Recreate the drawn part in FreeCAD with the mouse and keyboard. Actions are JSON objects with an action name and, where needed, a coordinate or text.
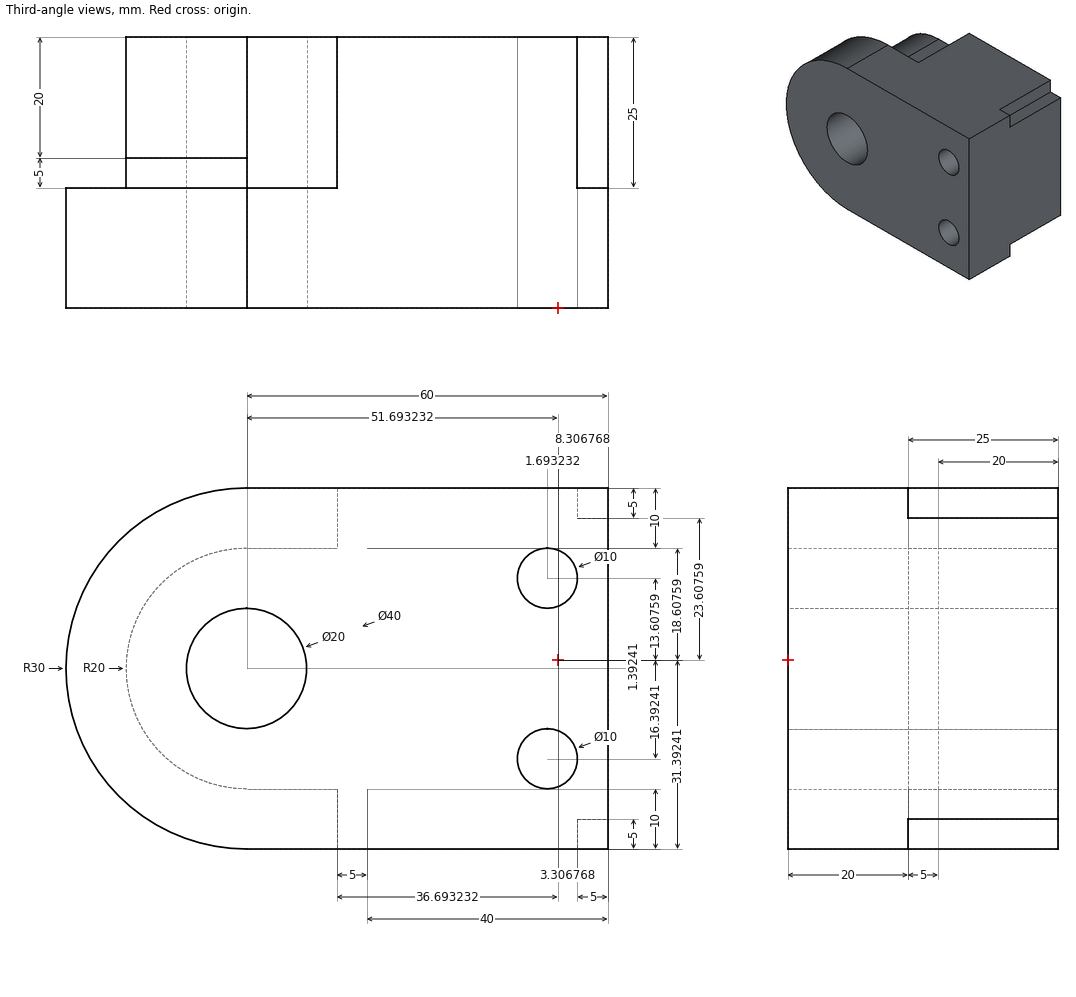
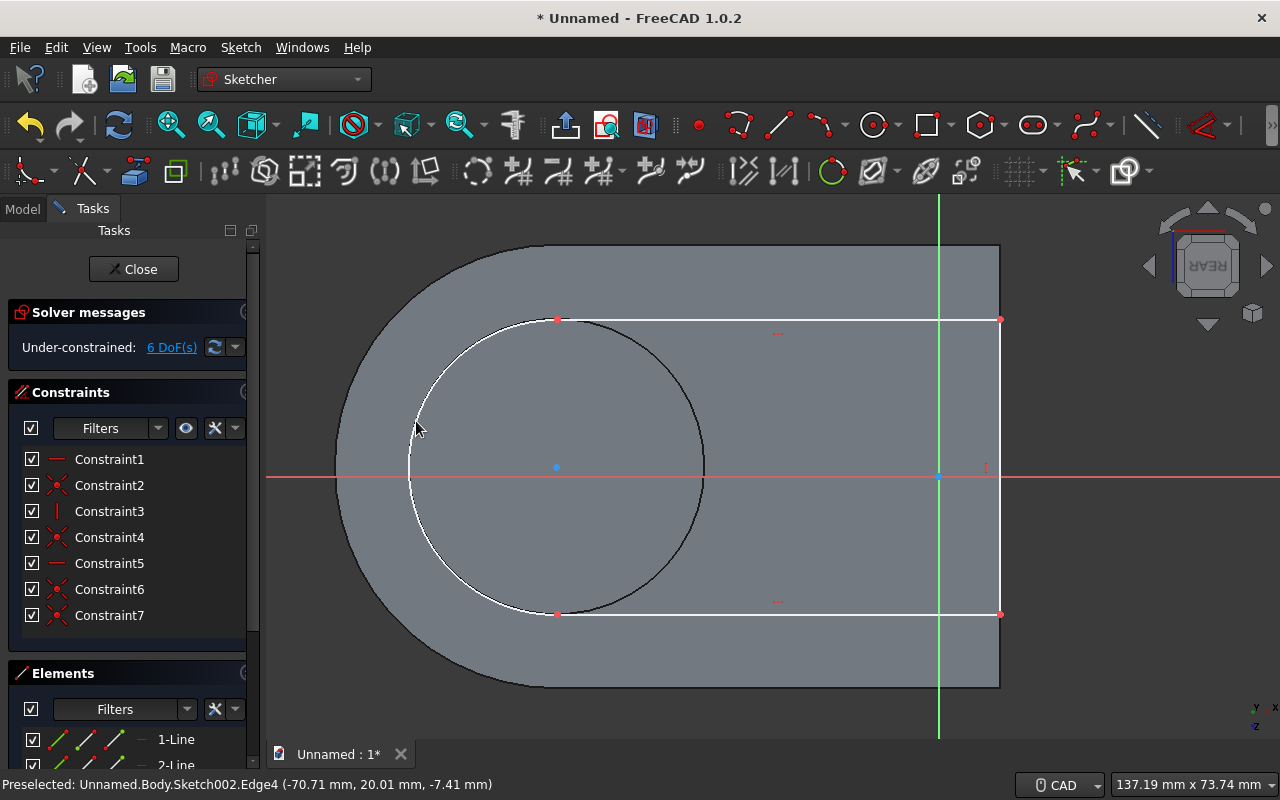
{"action": "left_click", "coordinate": [690, 615]}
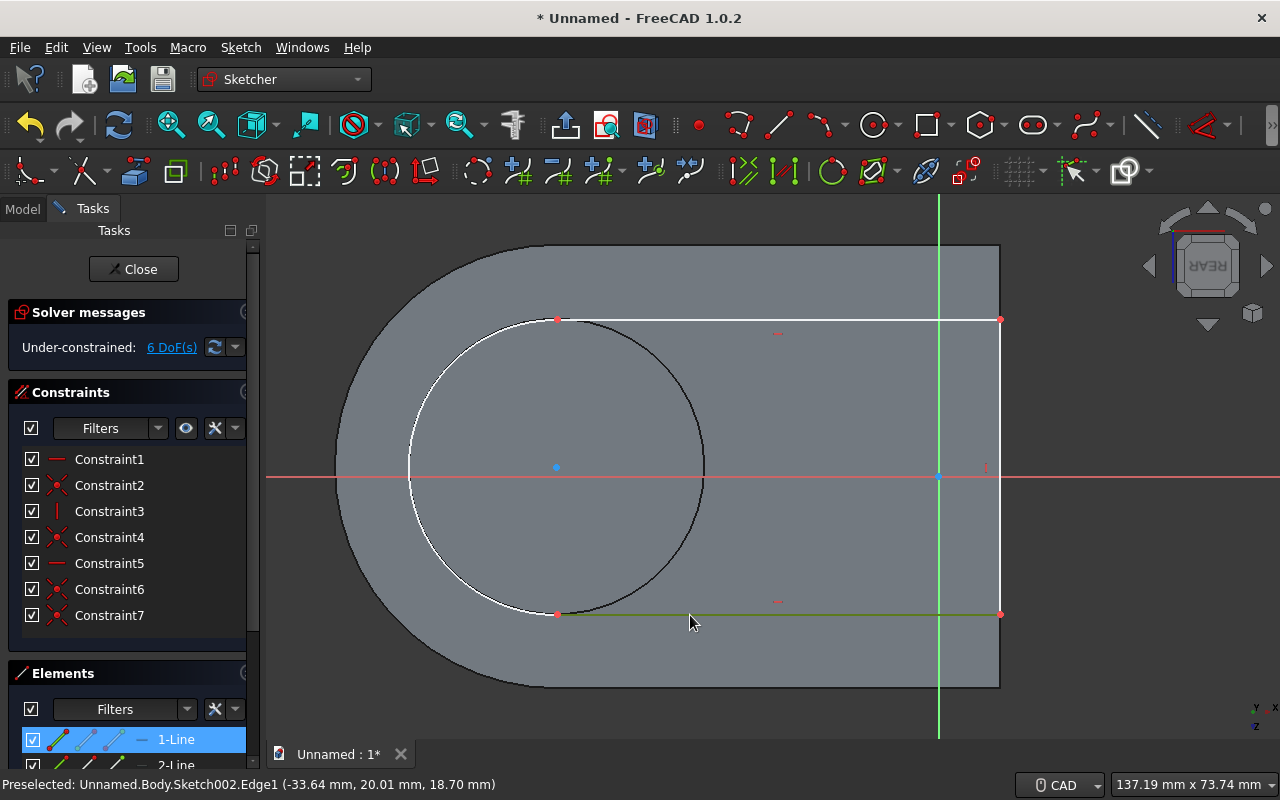
{"action": "left_click", "coordinate": [437, 381]}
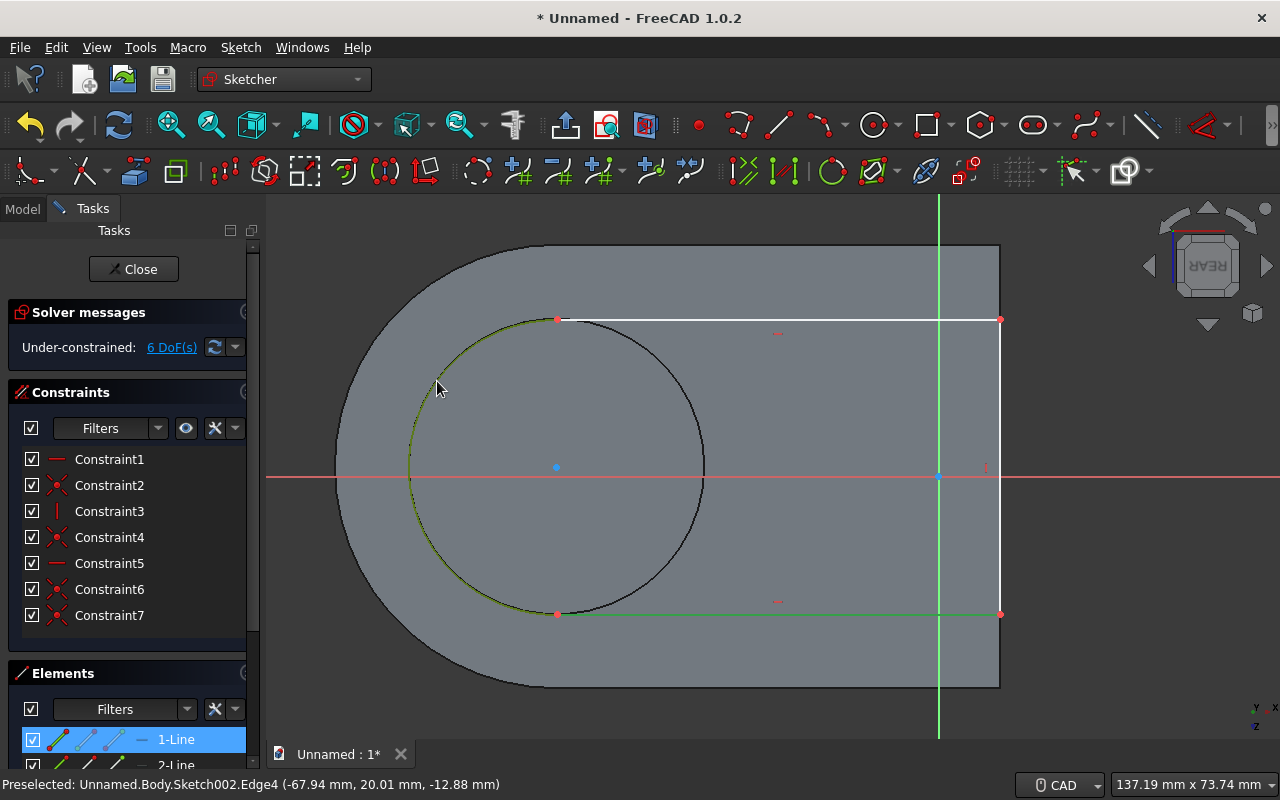
{"action": "key", "text": "t"}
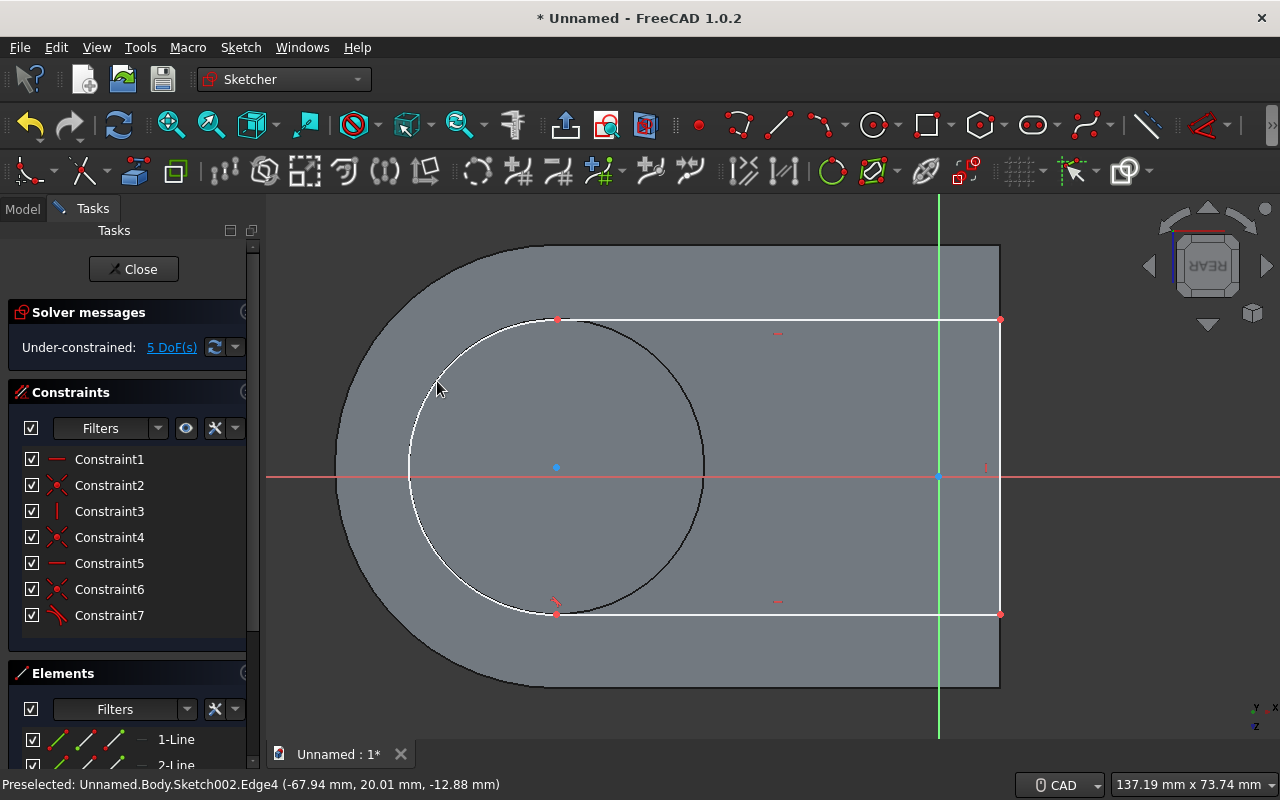
{"action": "left_click", "coordinate": [867, 320]}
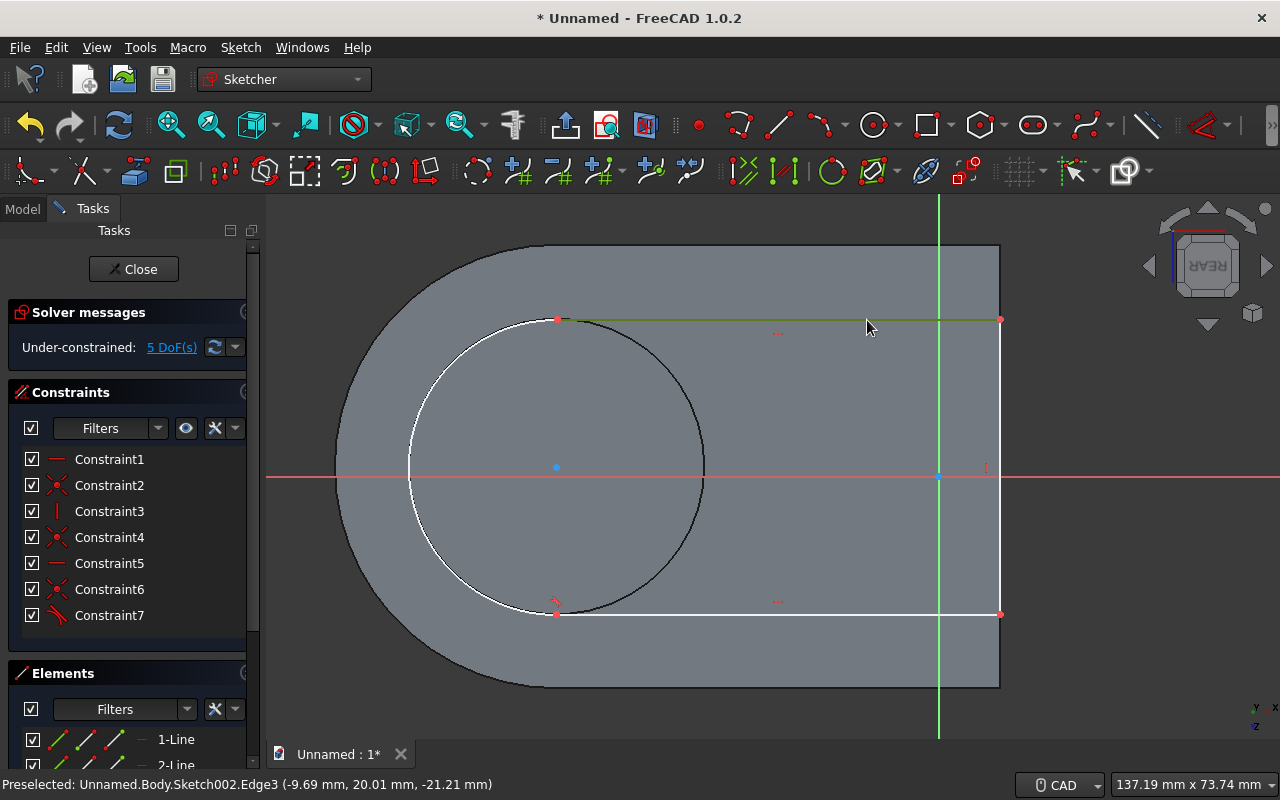
{"action": "left_click", "coordinate": [437, 380]}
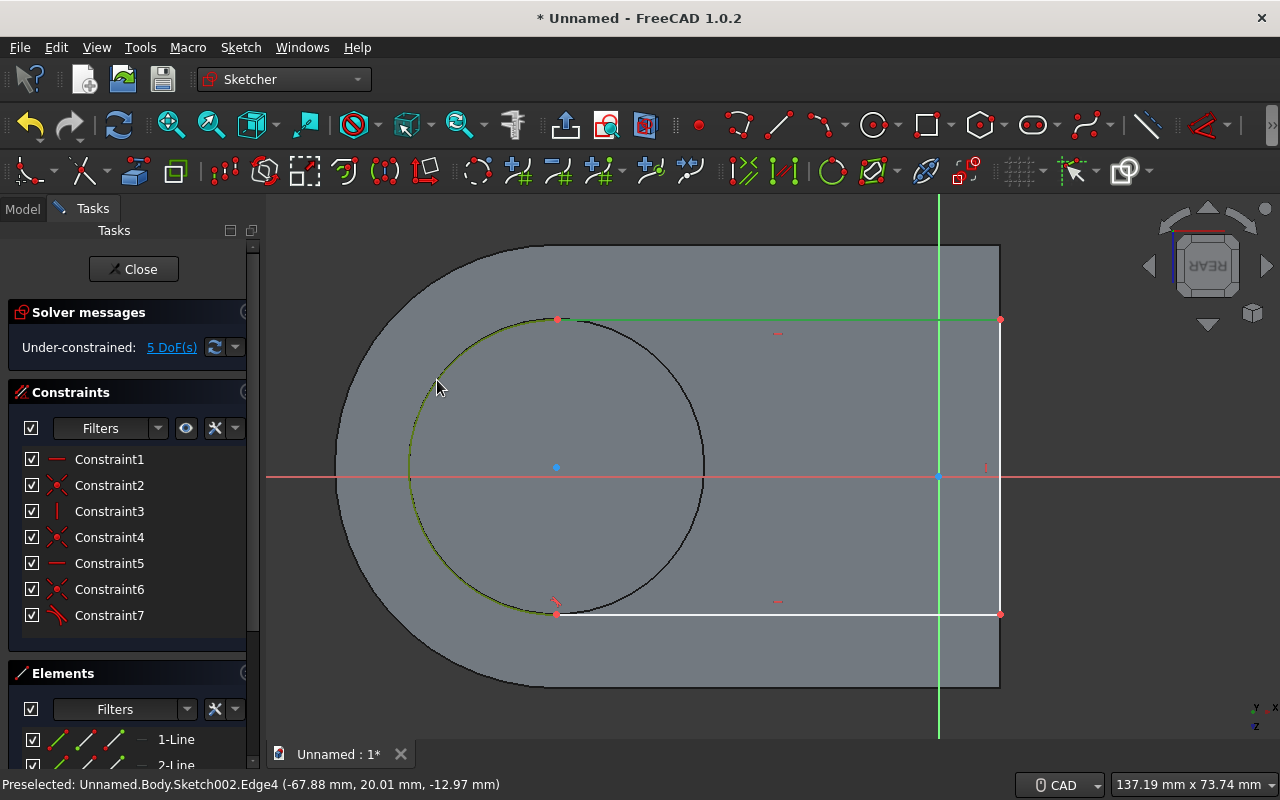
{"action": "key", "text": "t"}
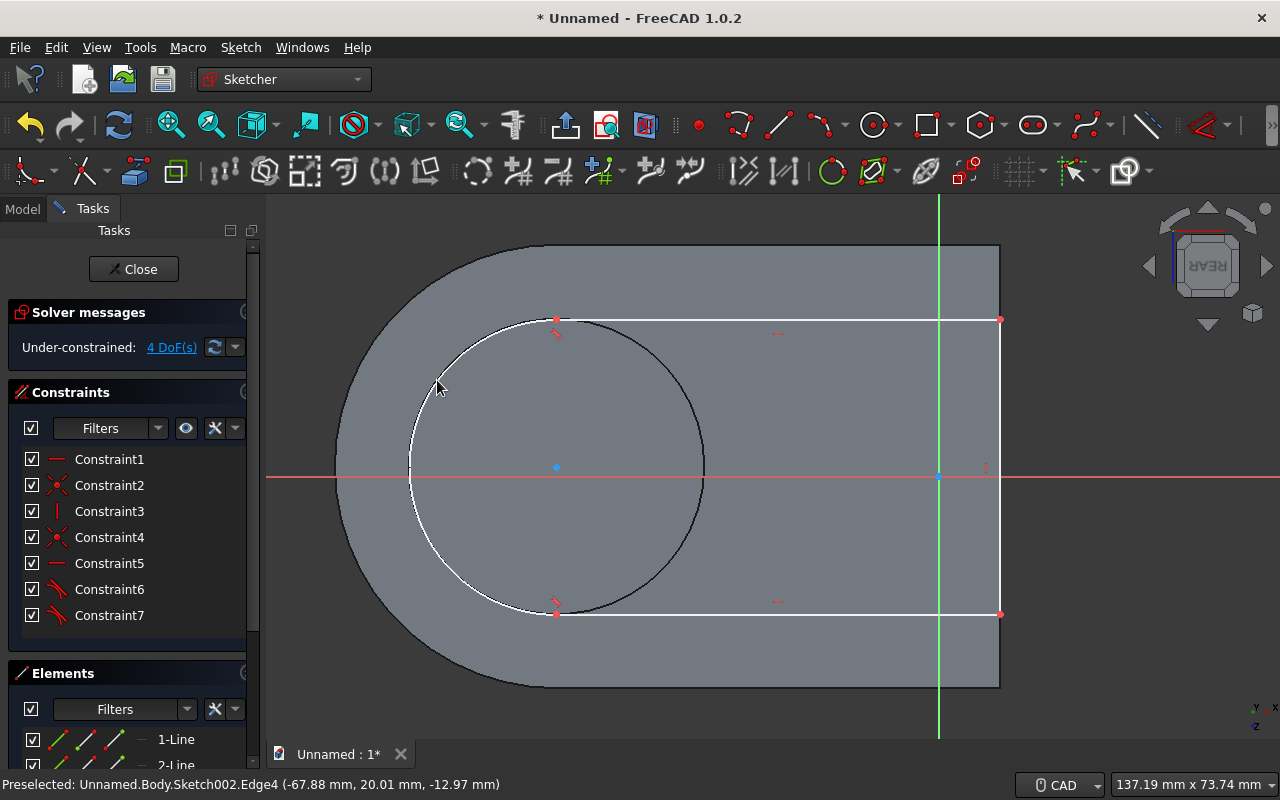
{"action": "key", "text": "d"}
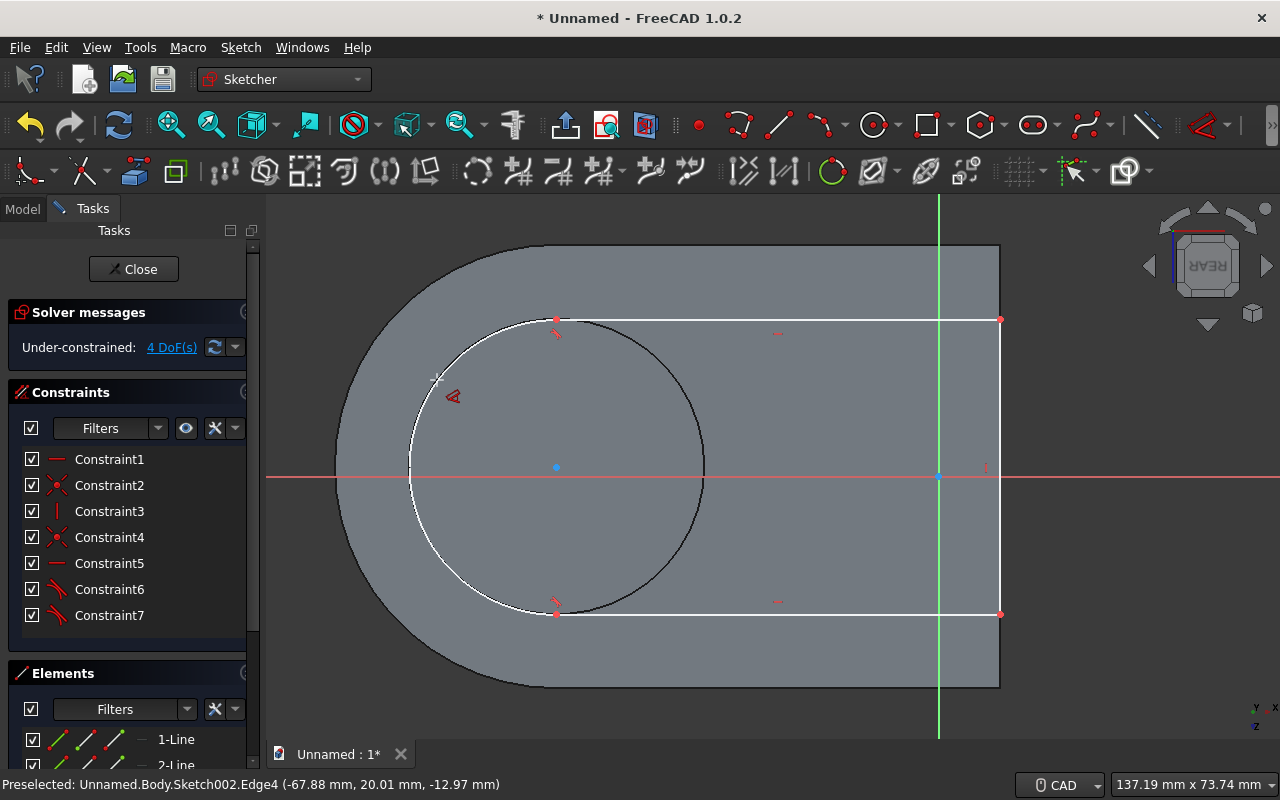
{"action": "left_click", "coordinate": [438, 381]}
{"action": "left_click", "coordinate": [412, 362]}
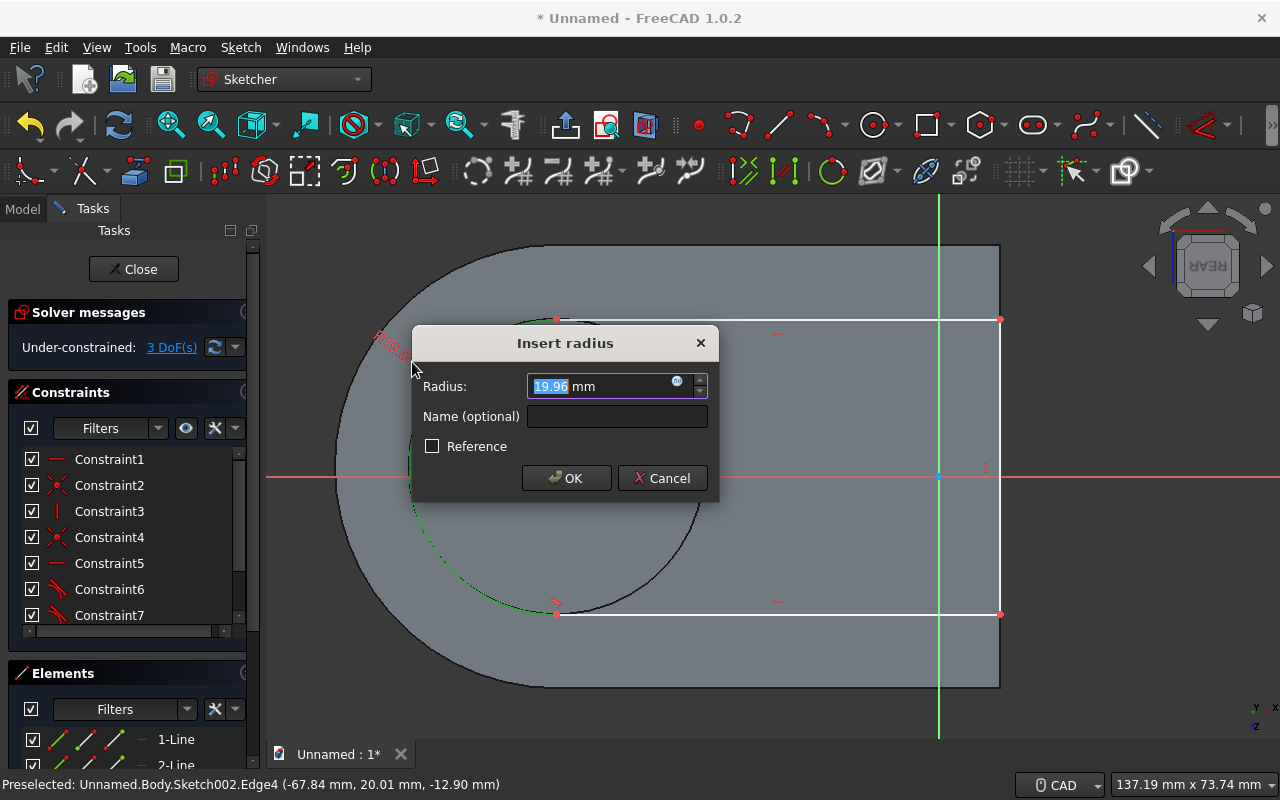
{"action": "type", "text": "20"}
{"action": "key", "text": "Return"}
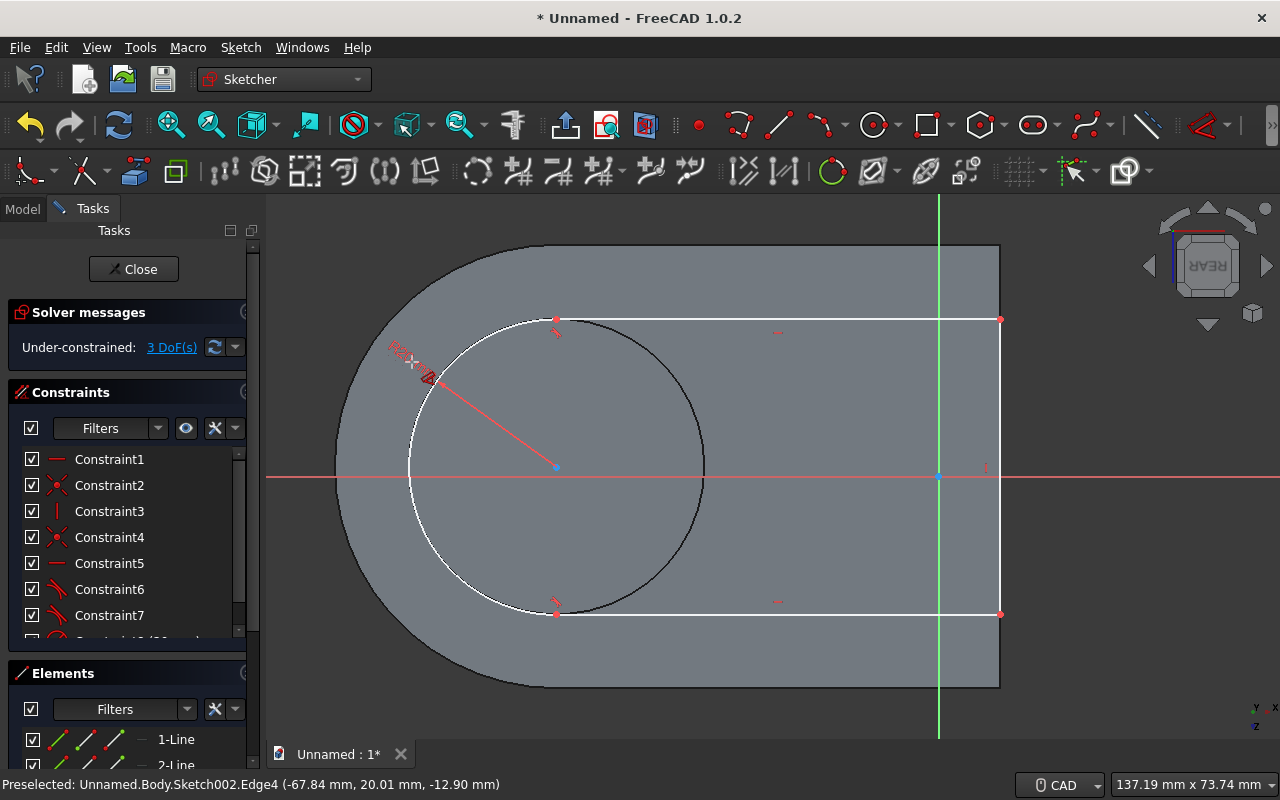
{"action": "left_click", "coordinate": [690, 615]}
{"action": "left_click", "coordinate": [778, 649]}